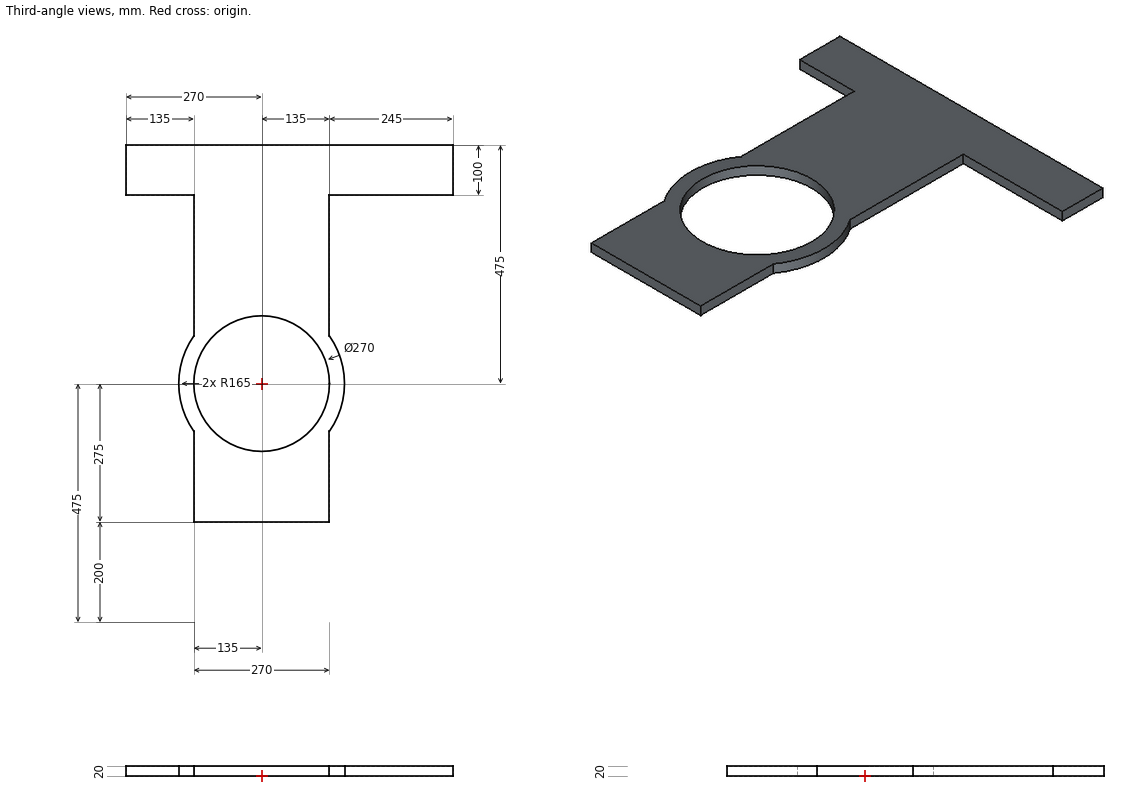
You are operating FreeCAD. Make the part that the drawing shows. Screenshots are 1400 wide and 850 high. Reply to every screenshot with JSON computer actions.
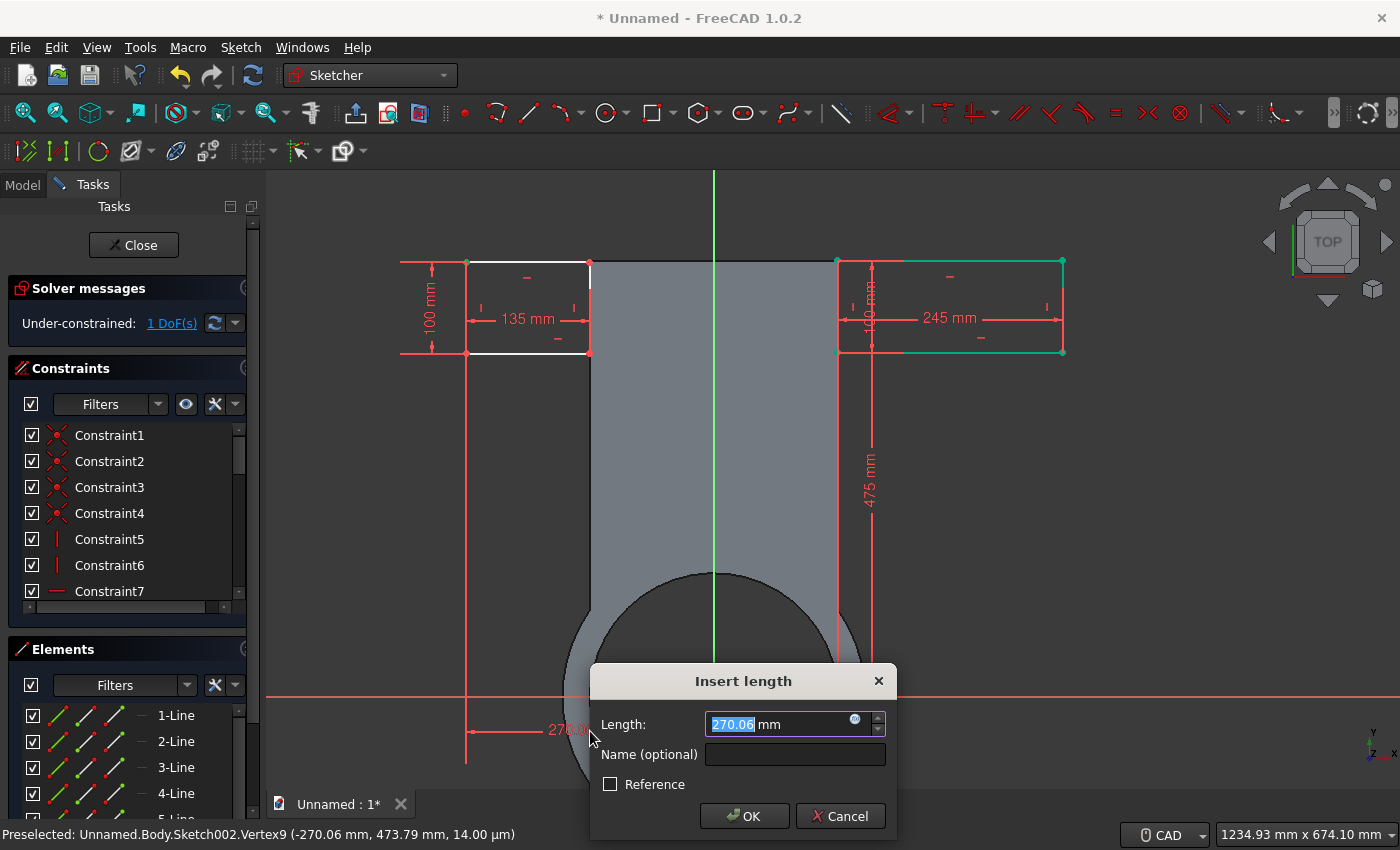
{"action": "type", "text": "270"}
{"action": "key", "text": "Return"}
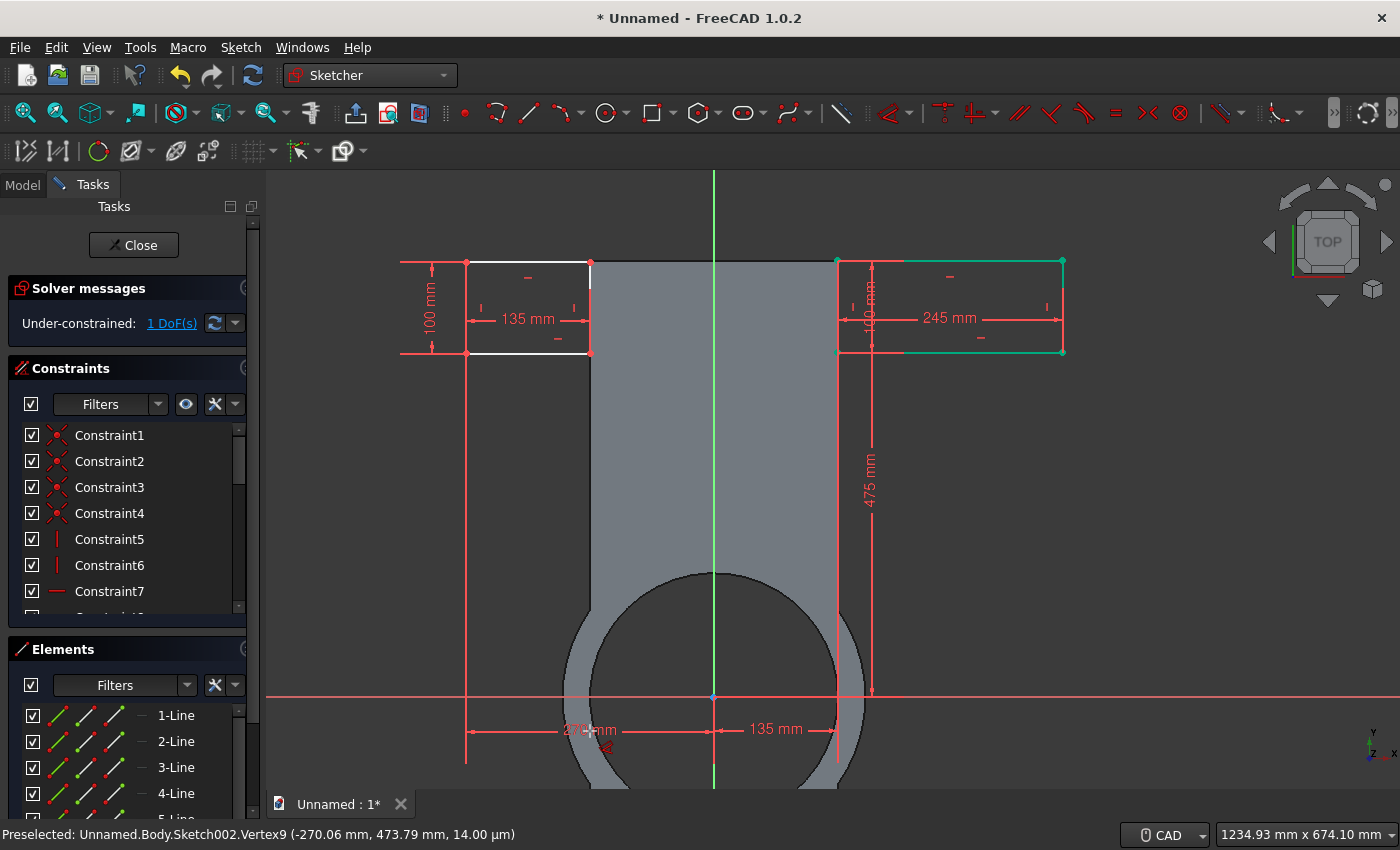
{"action": "left_click", "coordinate": [466, 262]}
{"action": "left_click", "coordinate": [432, 480]}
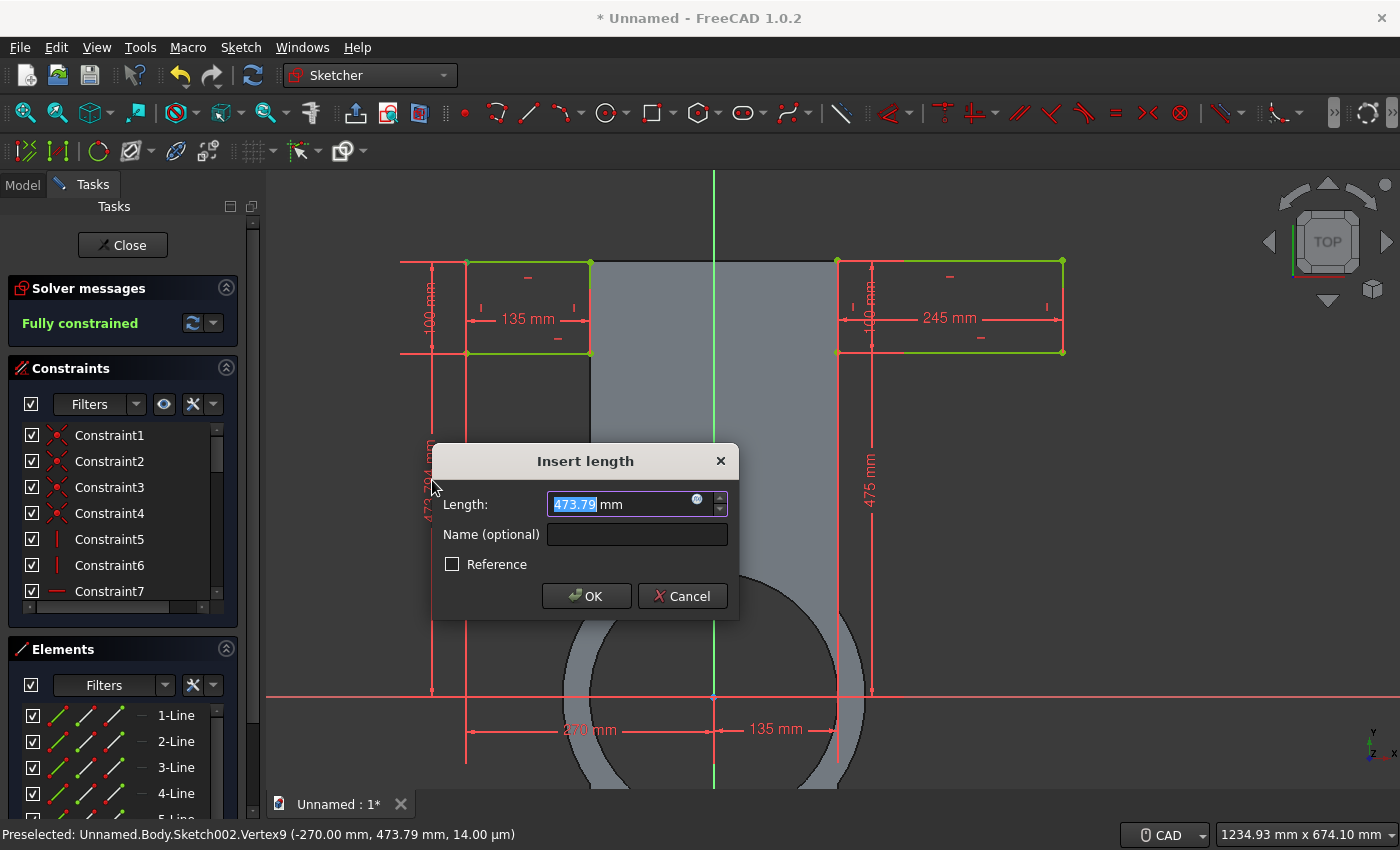
{"action": "type", "text": "475"}
{"action": "key", "text": "Return"}
{"action": "key", "text": "Escape"}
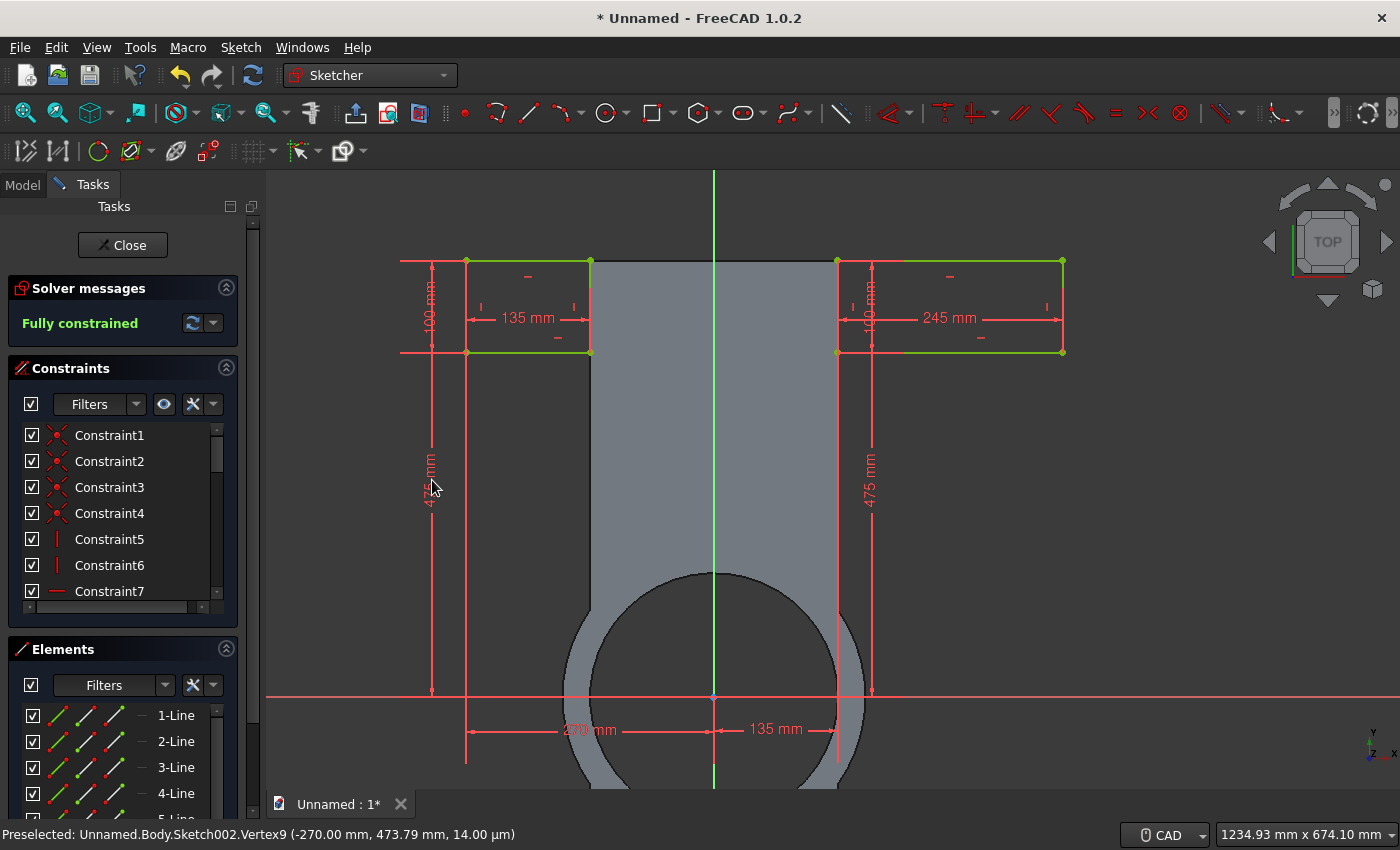
{"action": "left_click", "coordinate": [123, 245]}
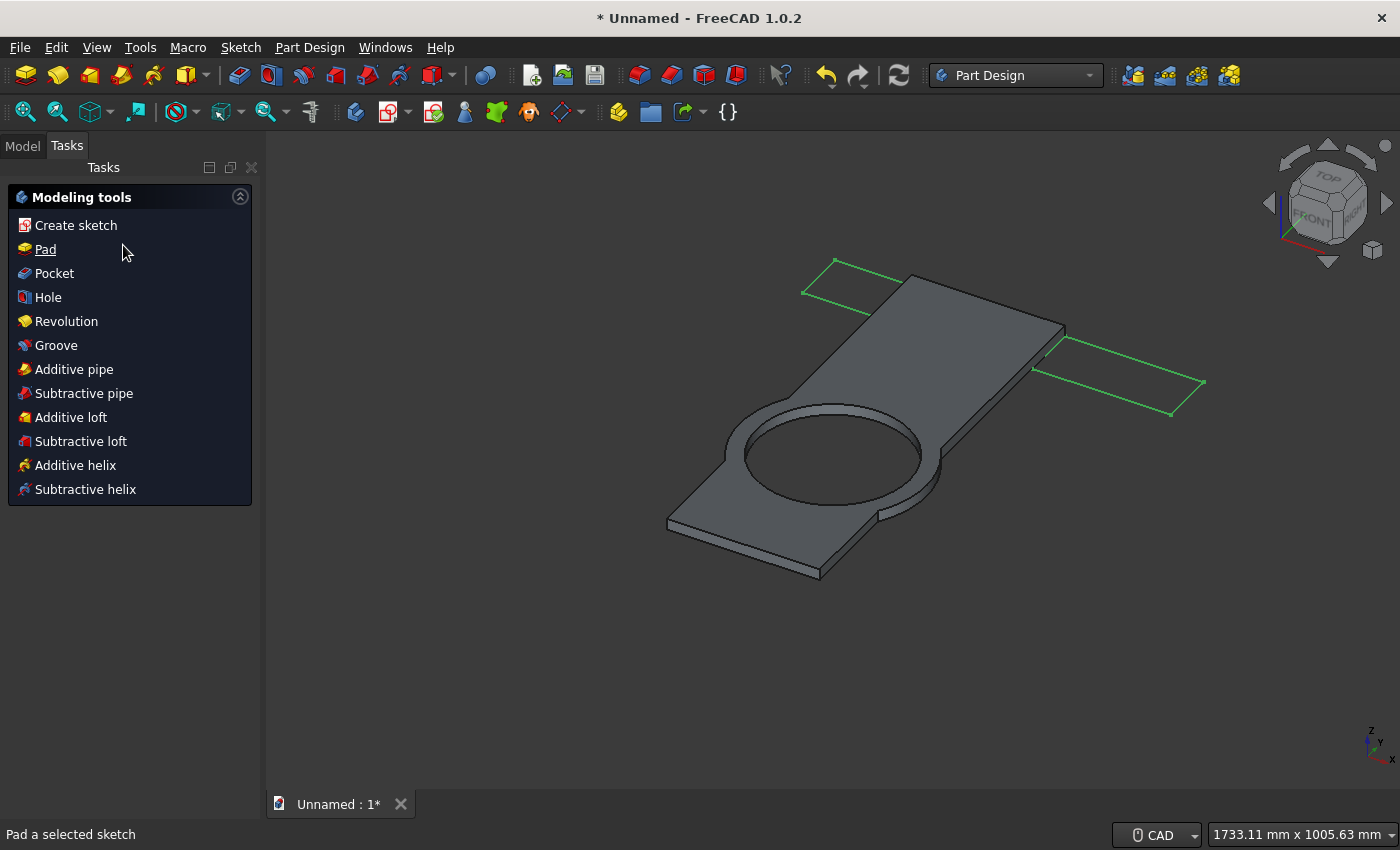
{"action": "left_click", "coordinate": [26, 76]}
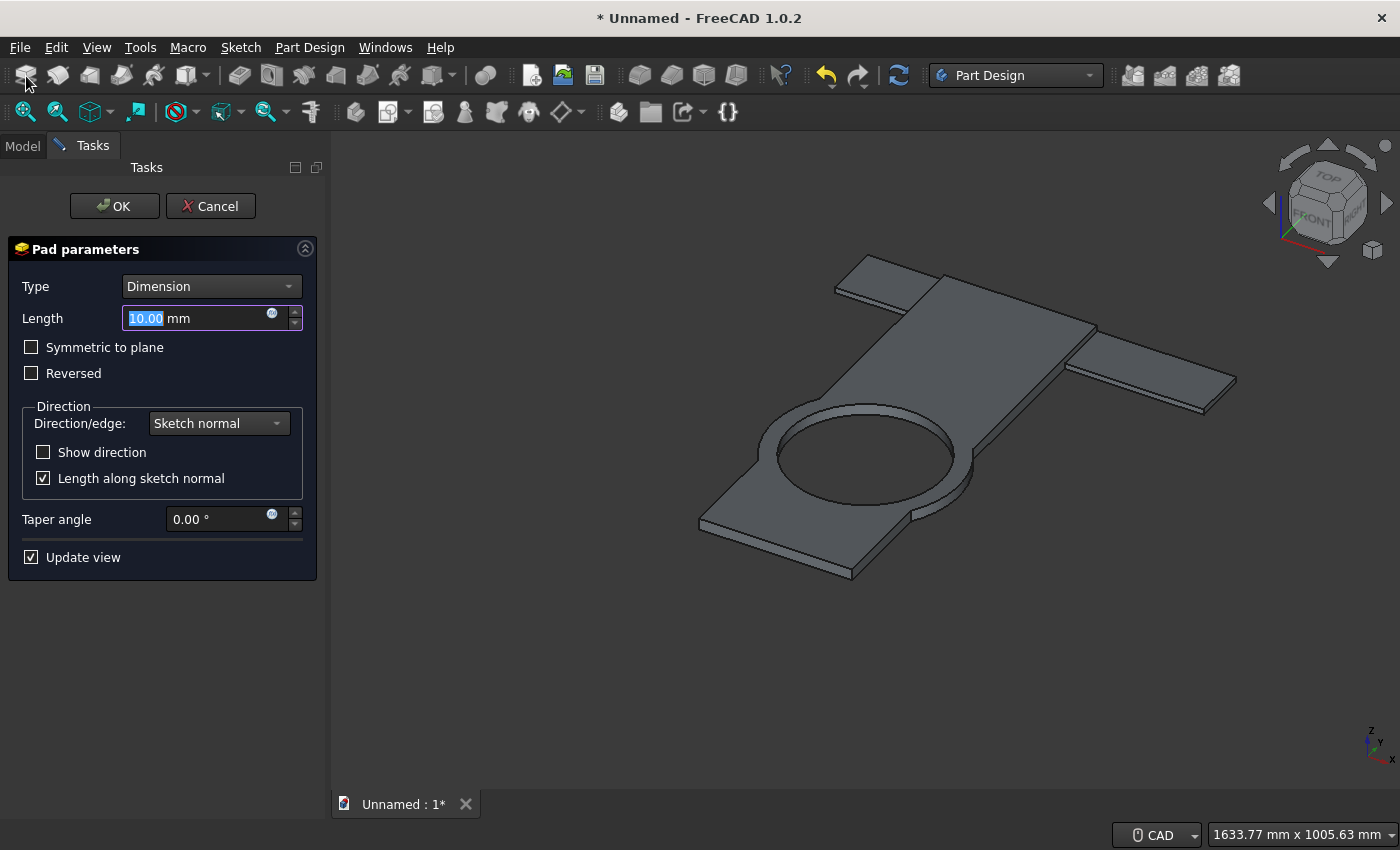
{"action": "type", "text": "20"}
{"action": "key", "text": "Tab"}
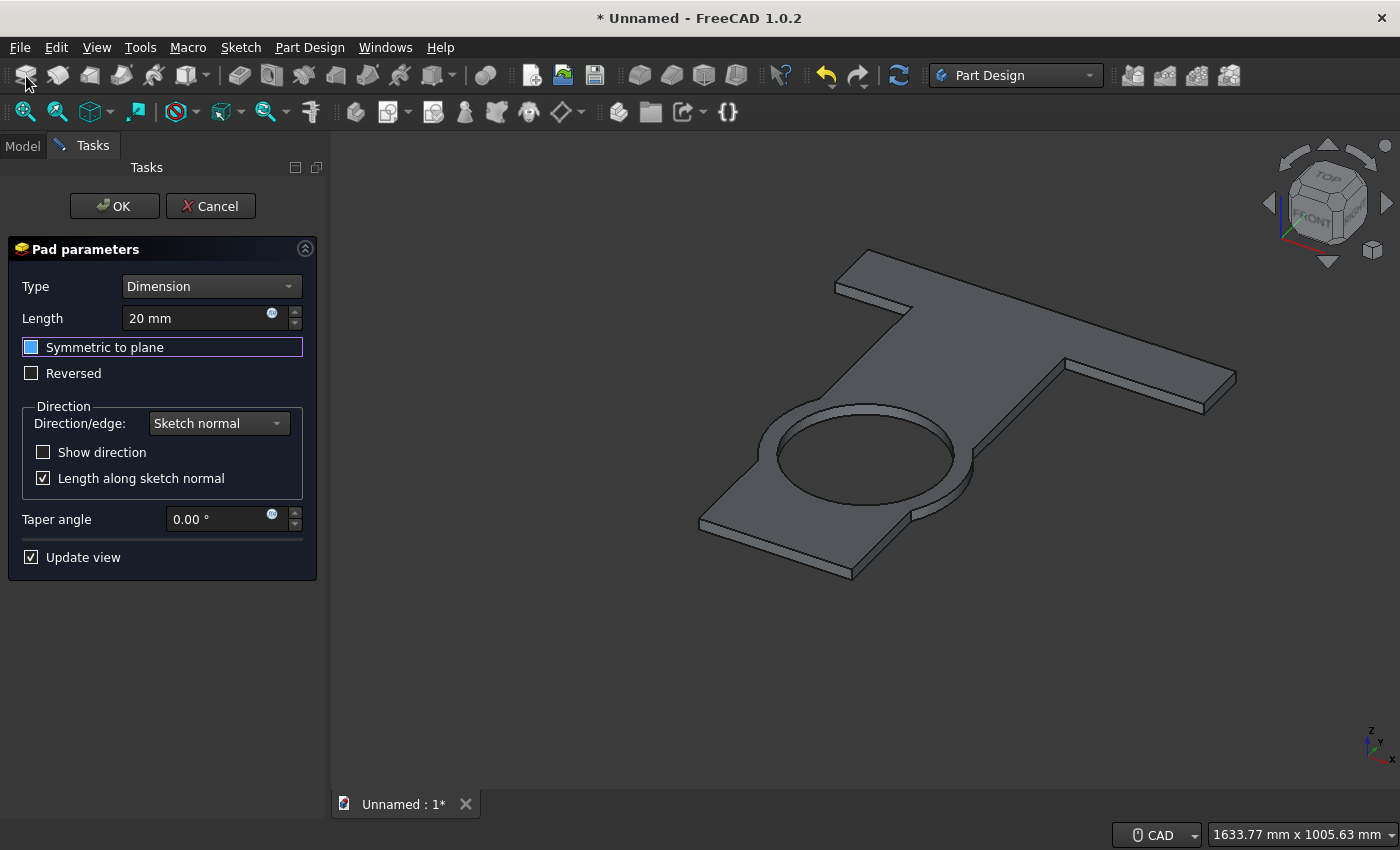
{"action": "left_click", "coordinate": [115, 206]}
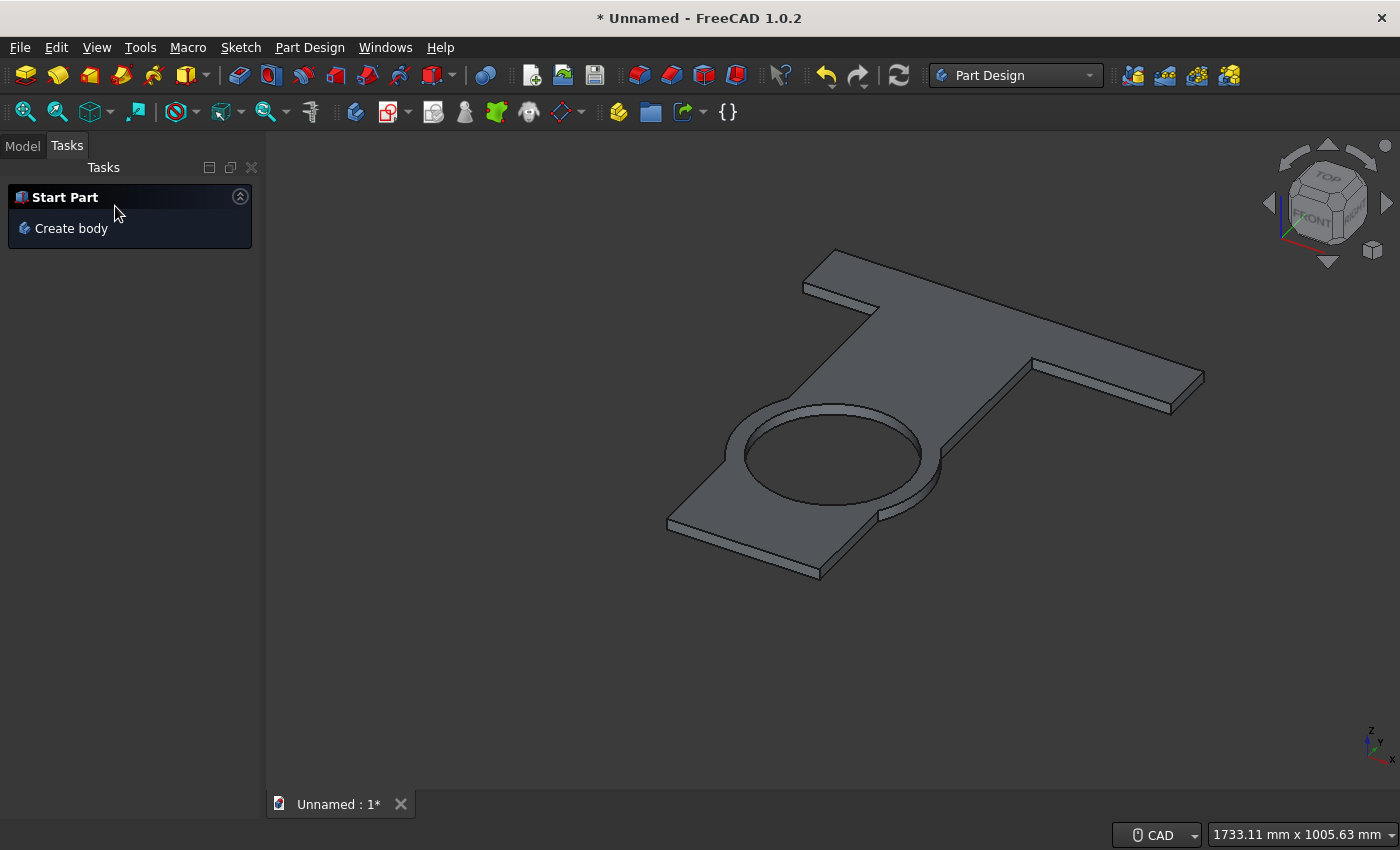
{"action": "key", "text": "0"}